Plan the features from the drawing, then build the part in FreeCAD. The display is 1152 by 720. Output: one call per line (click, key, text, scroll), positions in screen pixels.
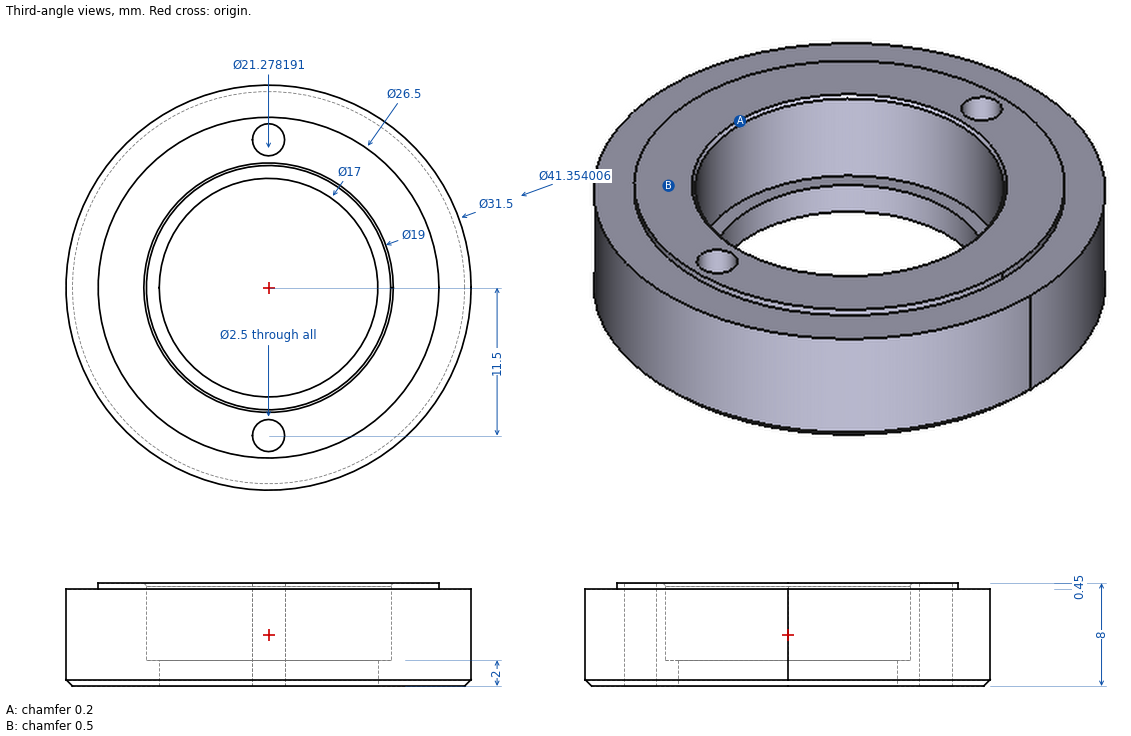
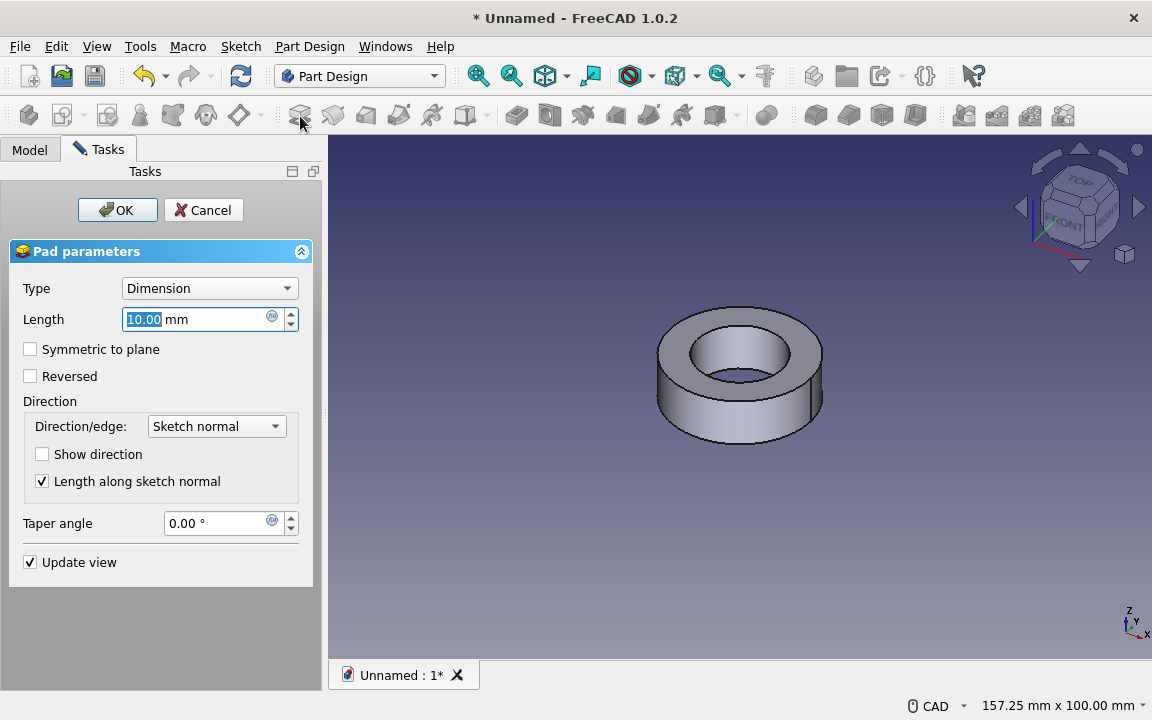
text(8)
key(Tab)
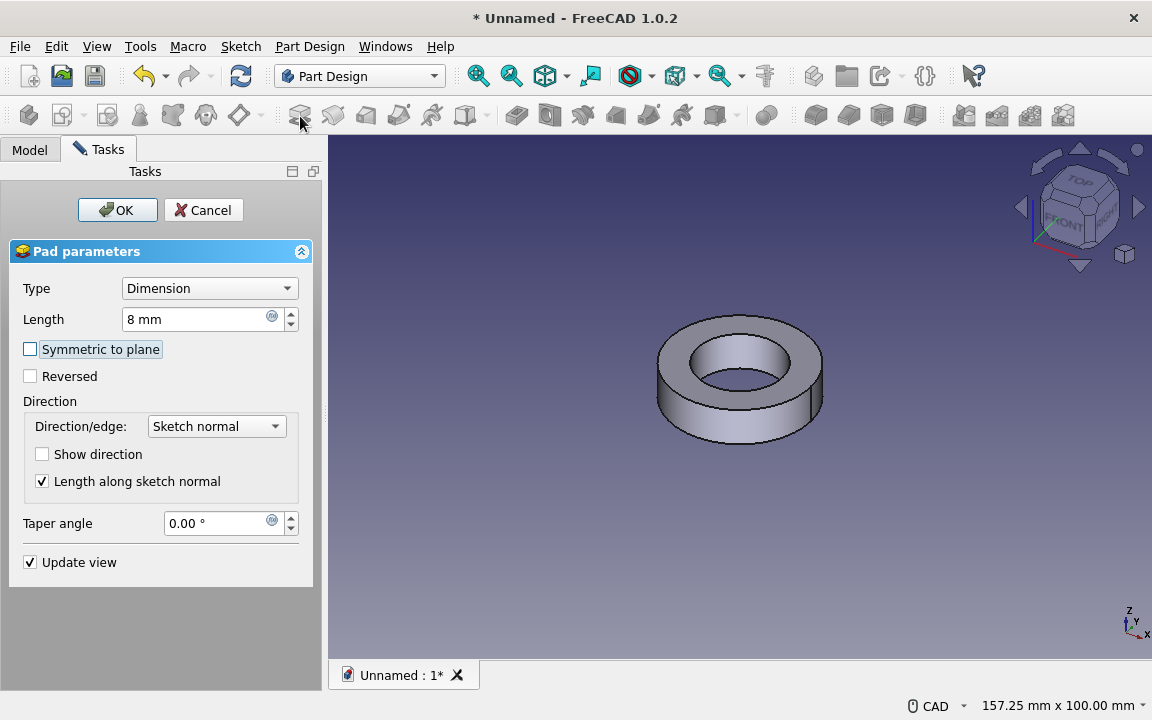
click(31, 349)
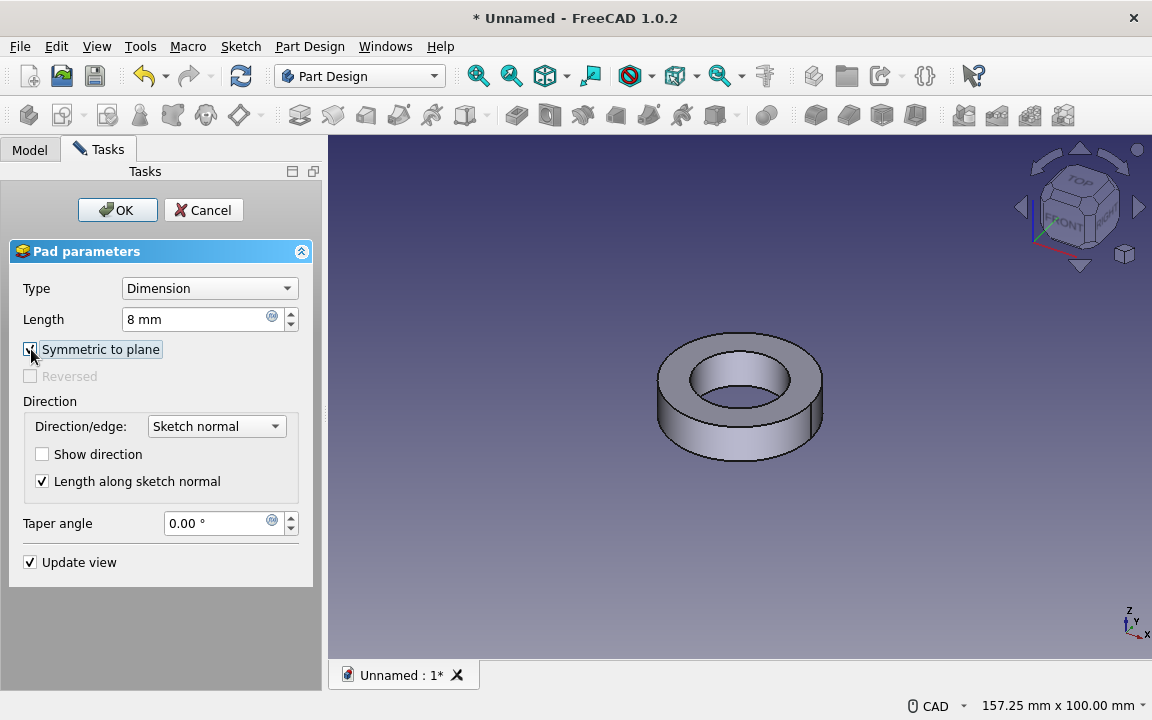
click(118, 210)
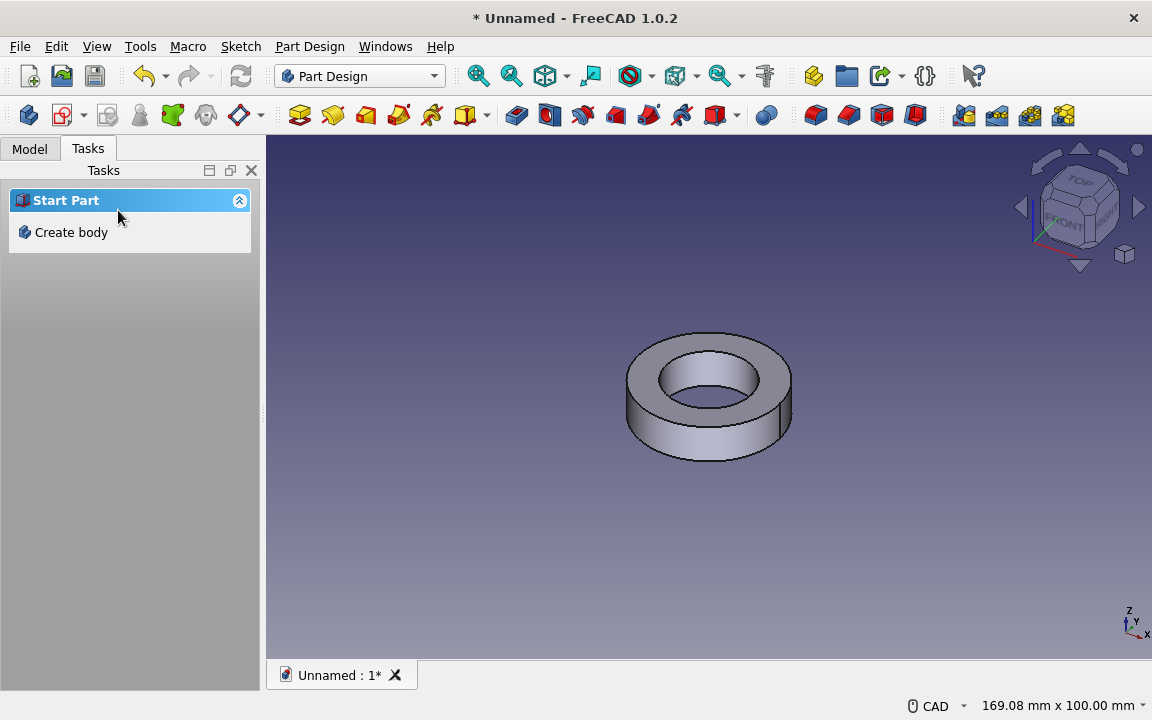
click(479, 76)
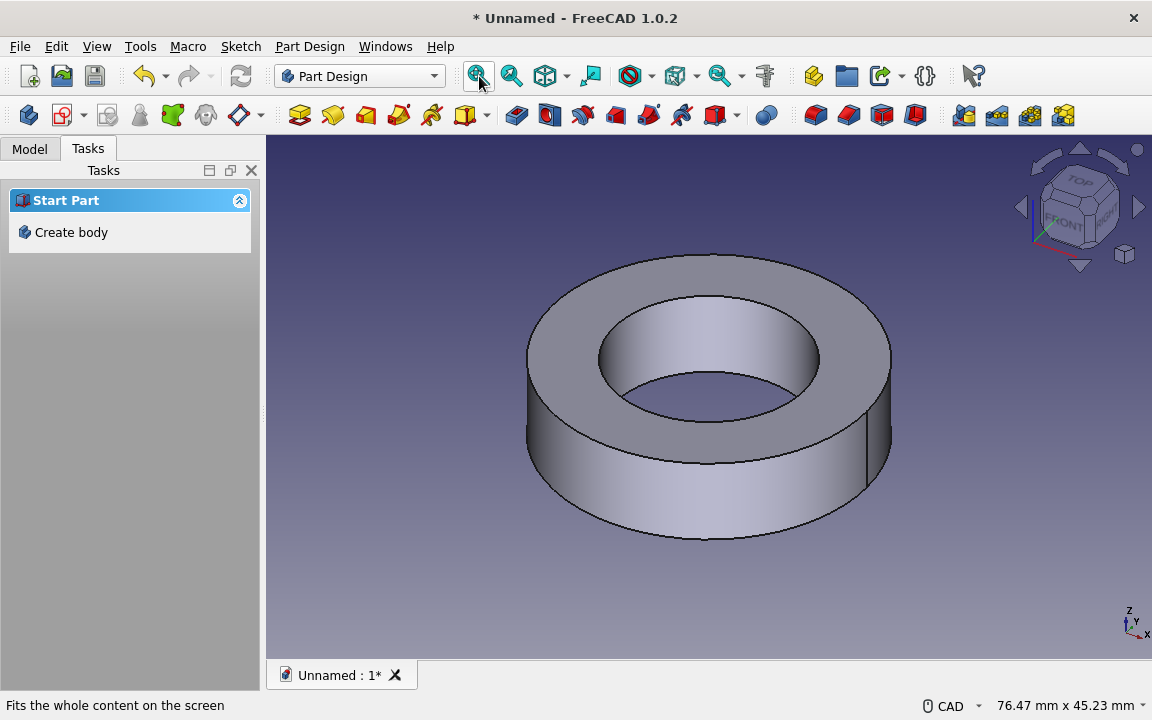
key(5)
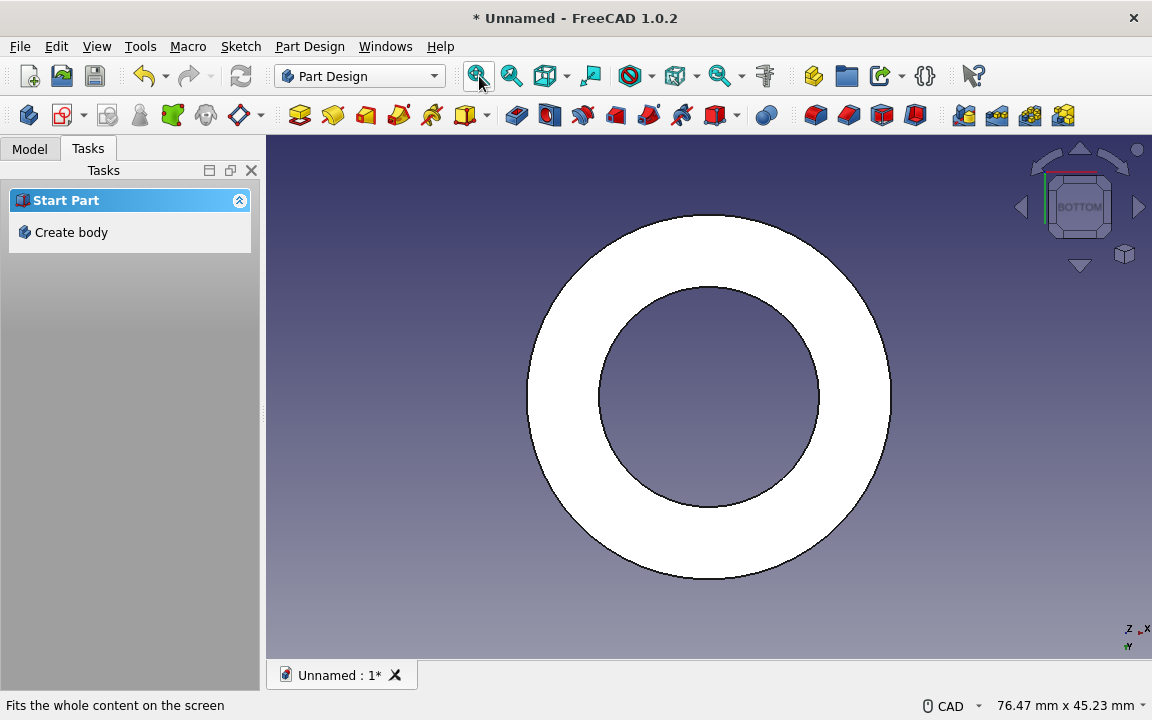
click(605, 292)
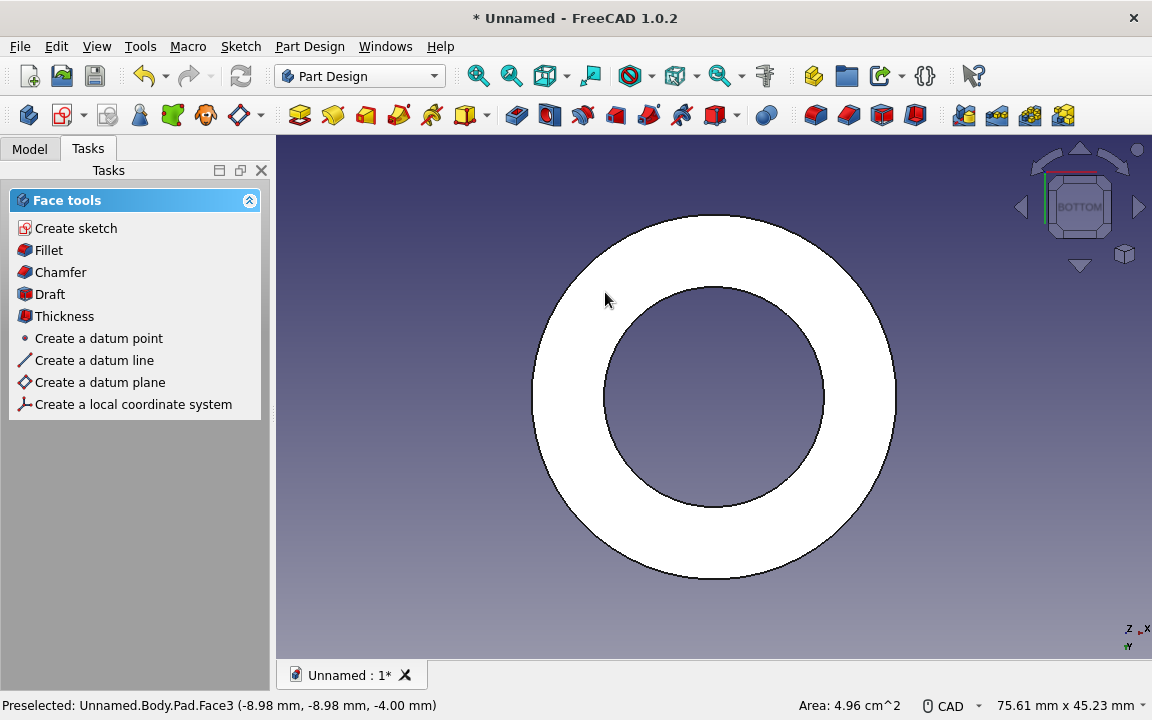
click(62, 116)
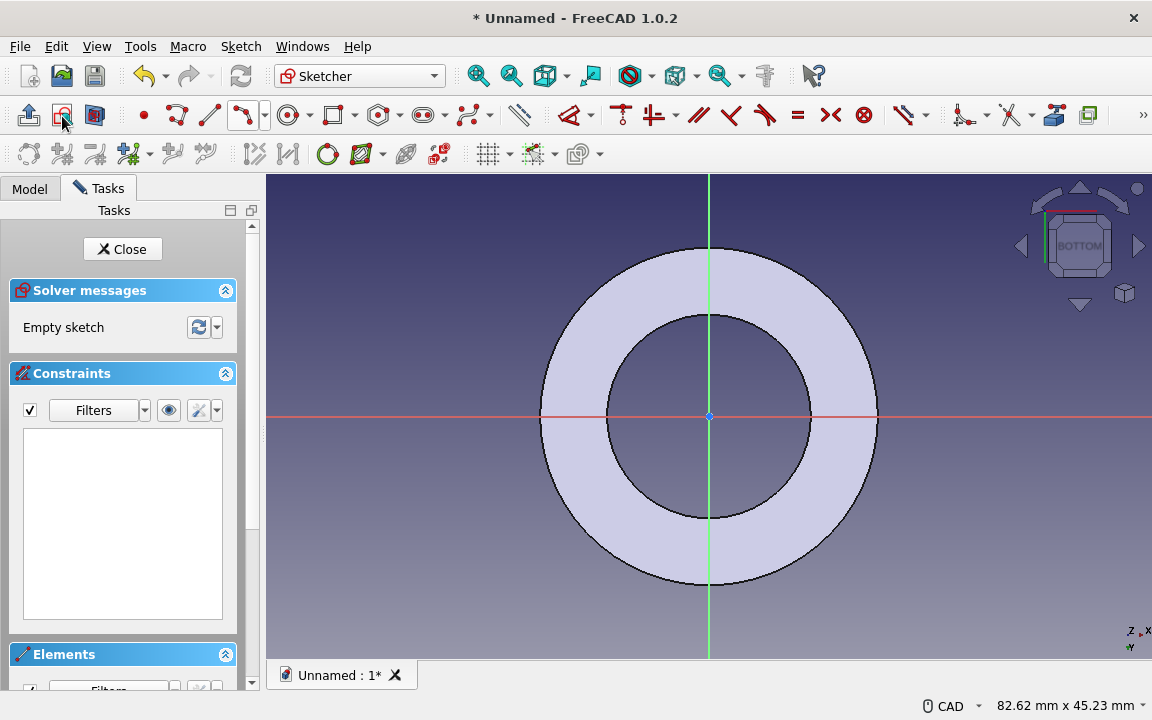
click(288, 116)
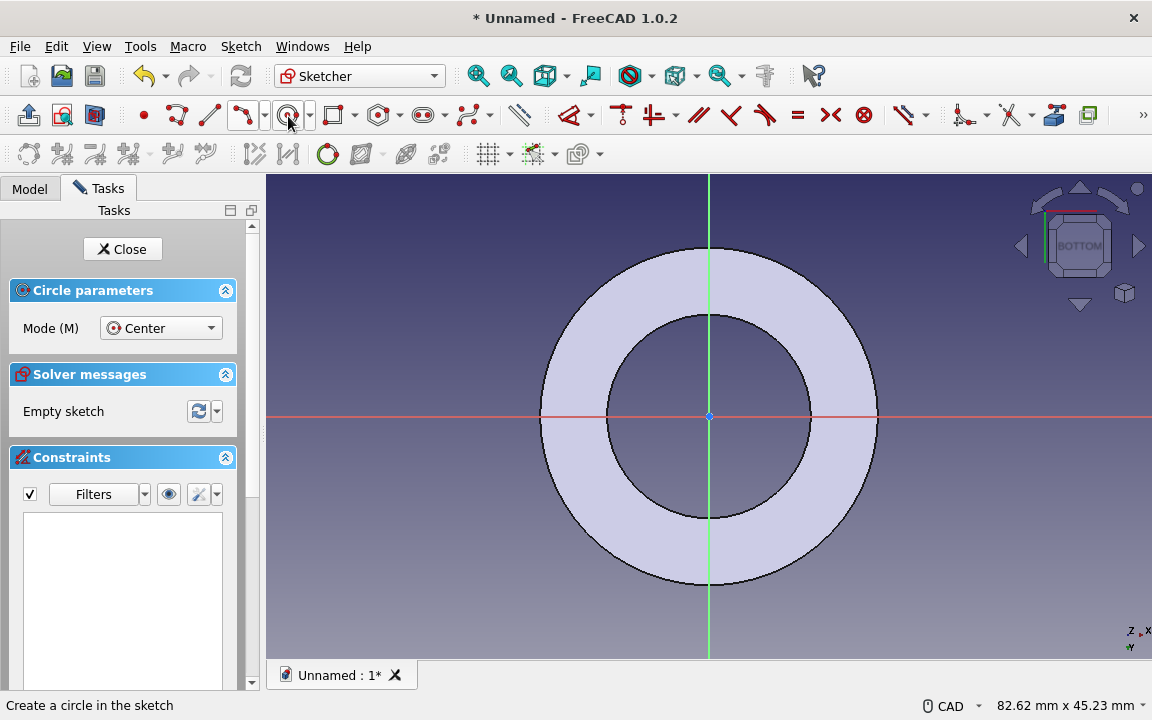
click(709, 416)
move(790, 336)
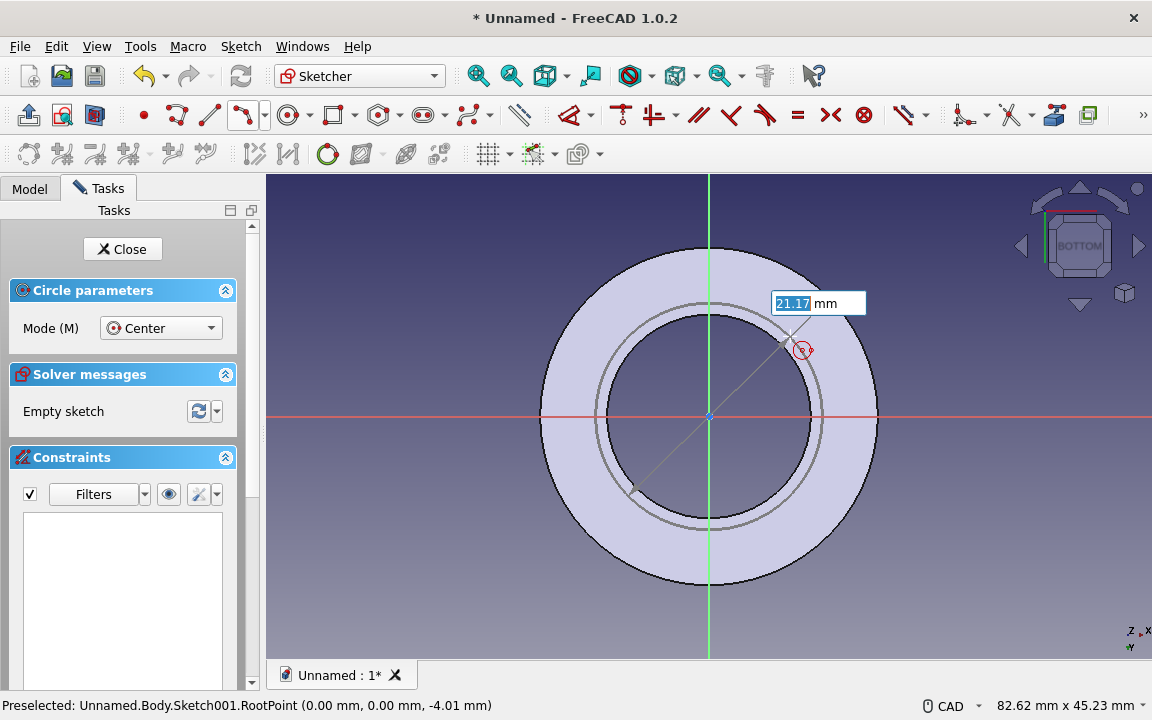
text(21.278191)
key(Return)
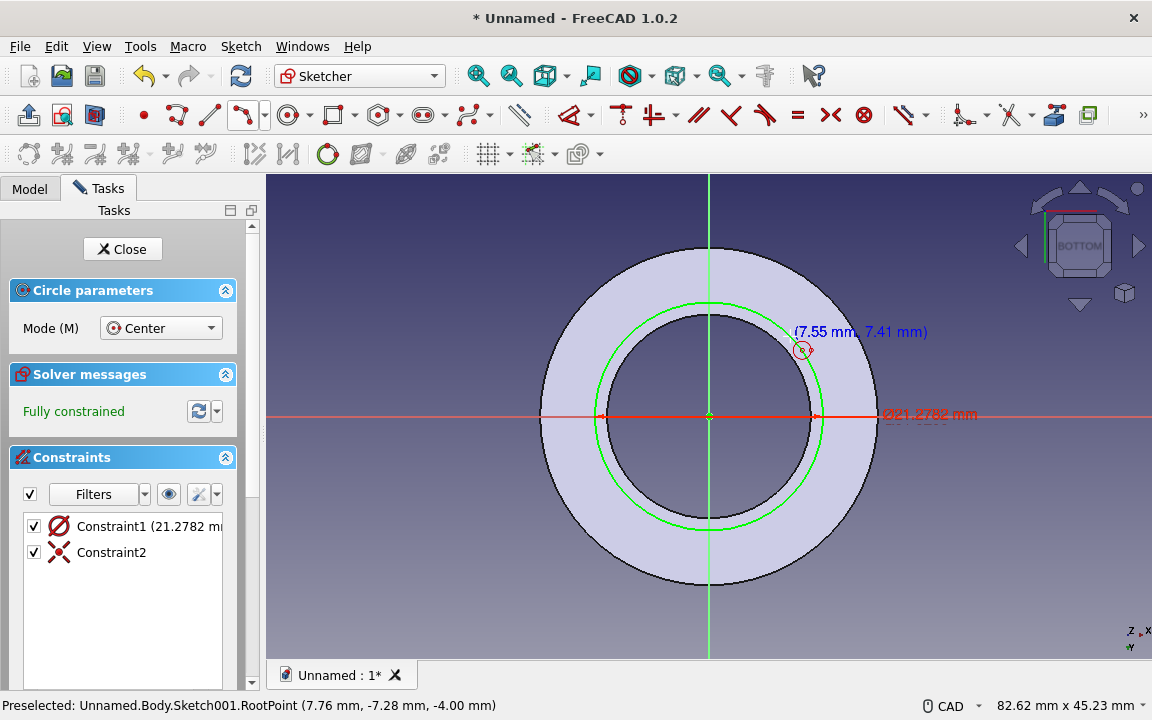
click(709, 416)
move(773, 352)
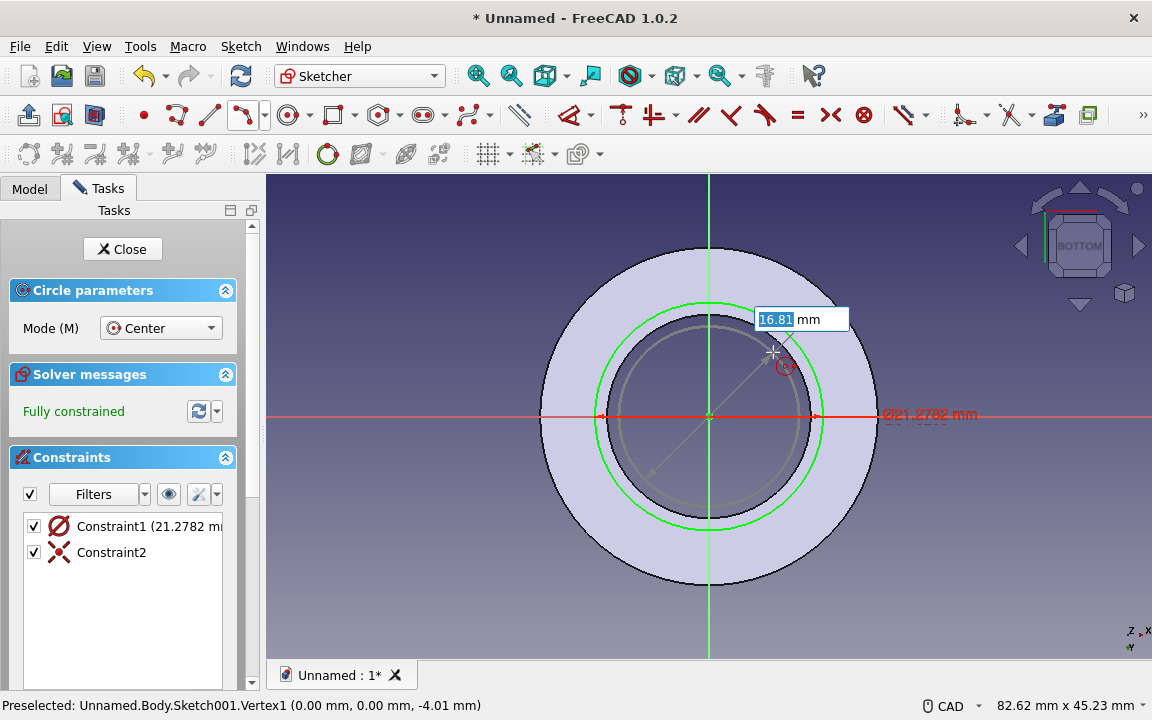
text(17)
key(Return)
key(Escape)